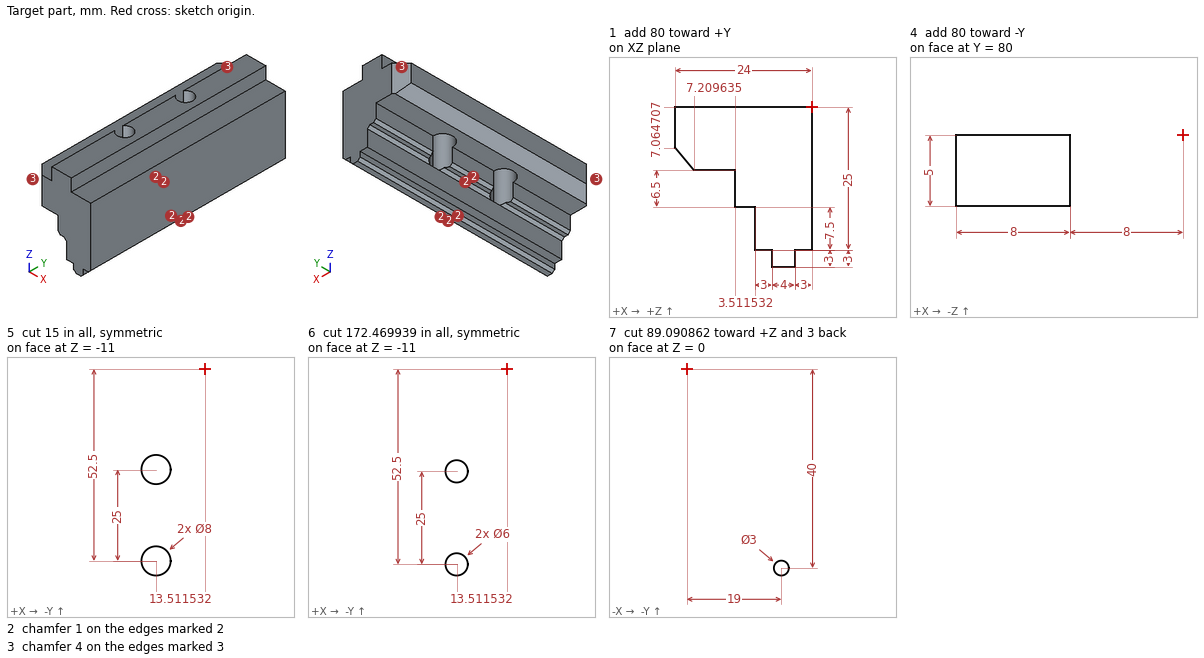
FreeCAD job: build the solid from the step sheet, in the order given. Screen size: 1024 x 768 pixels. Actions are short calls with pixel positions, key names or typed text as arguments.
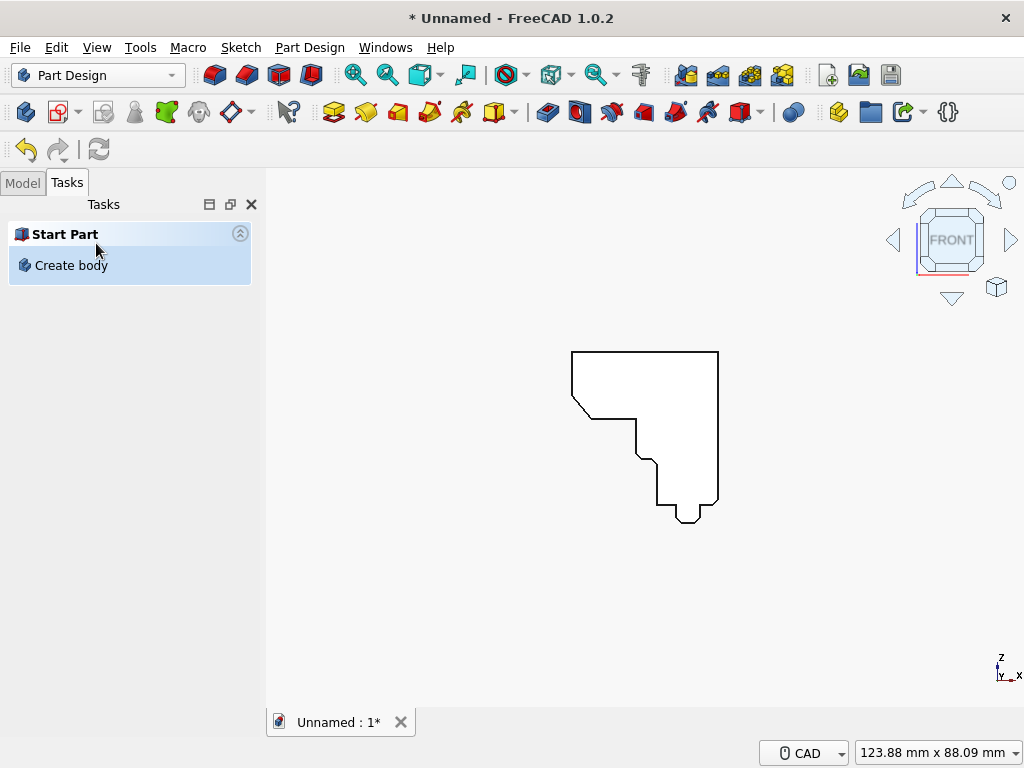
click(572, 372)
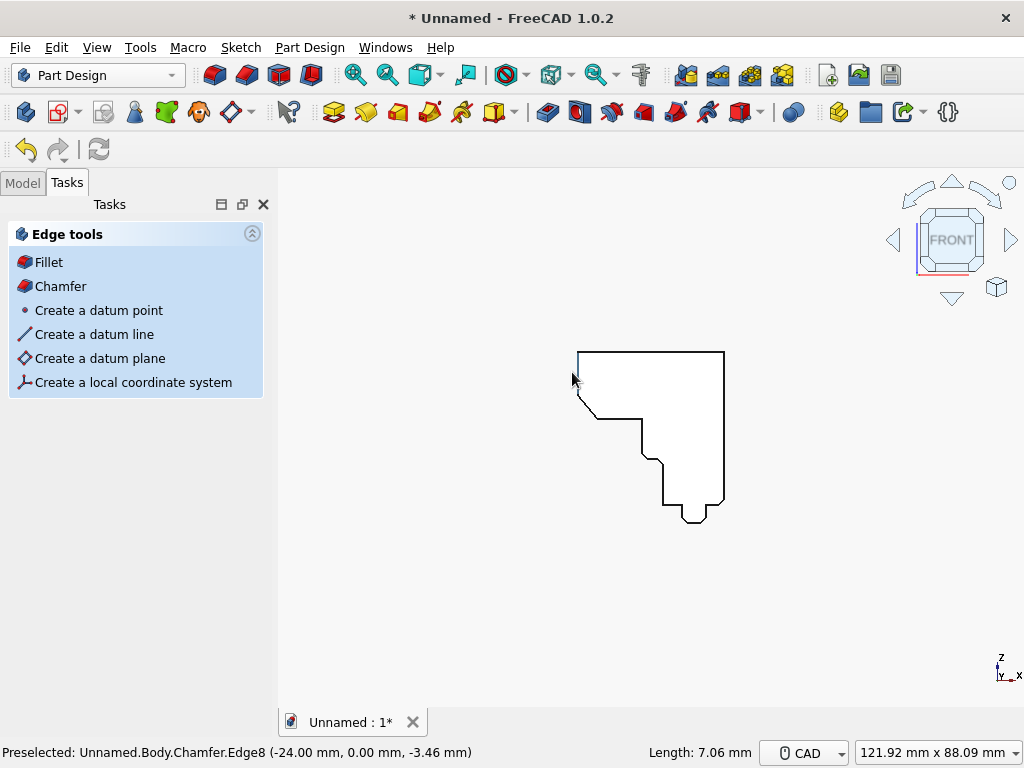
key(3)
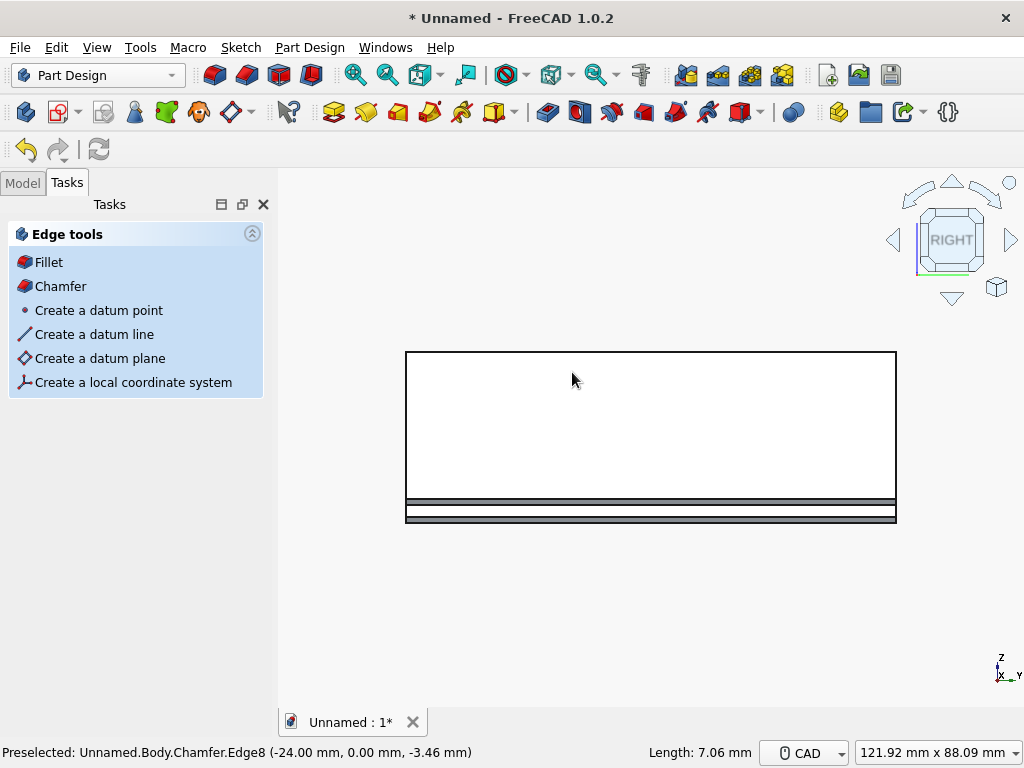
key(5)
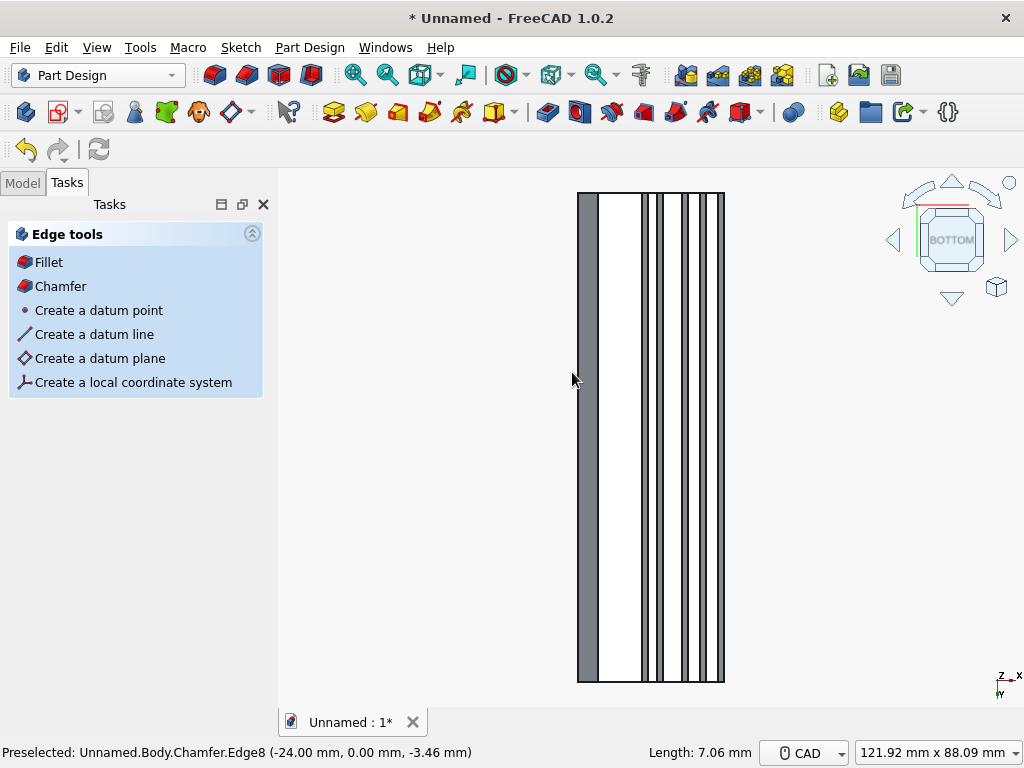
key(4)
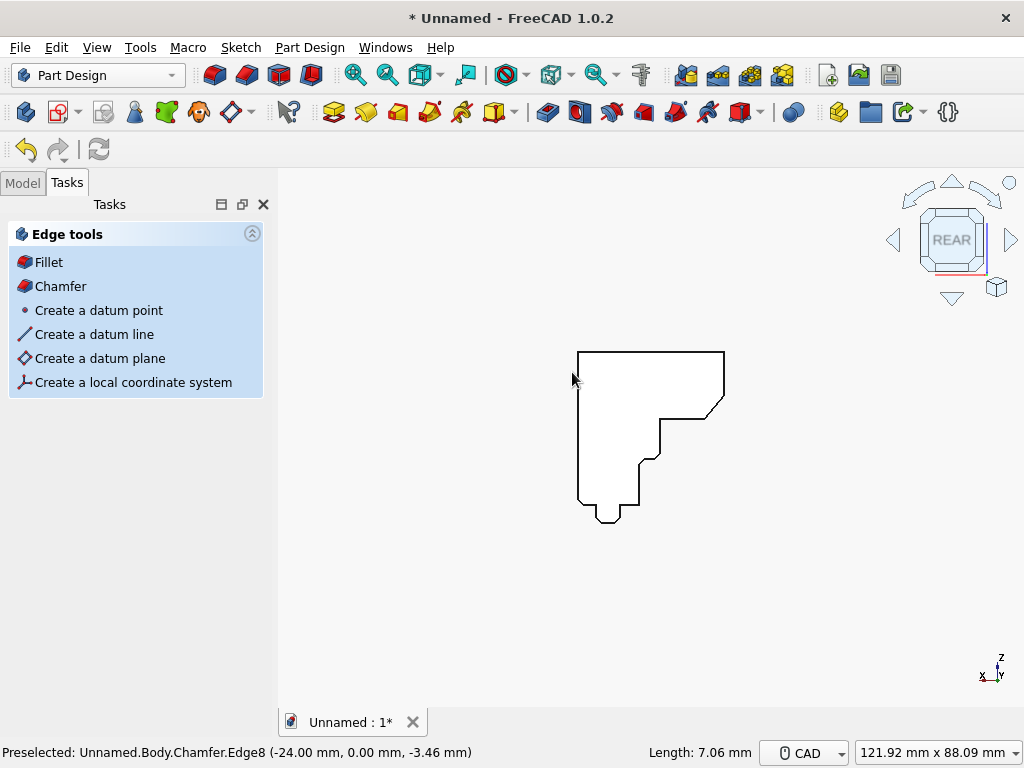
key(v)
key(f)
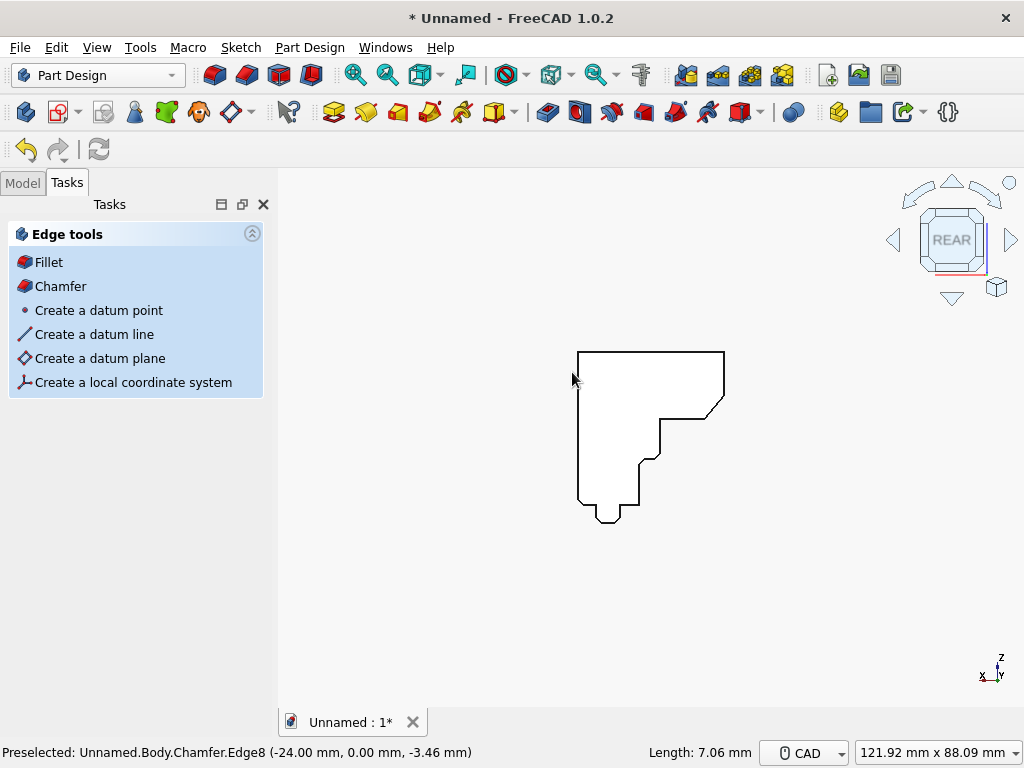
click(724, 372, ctrl)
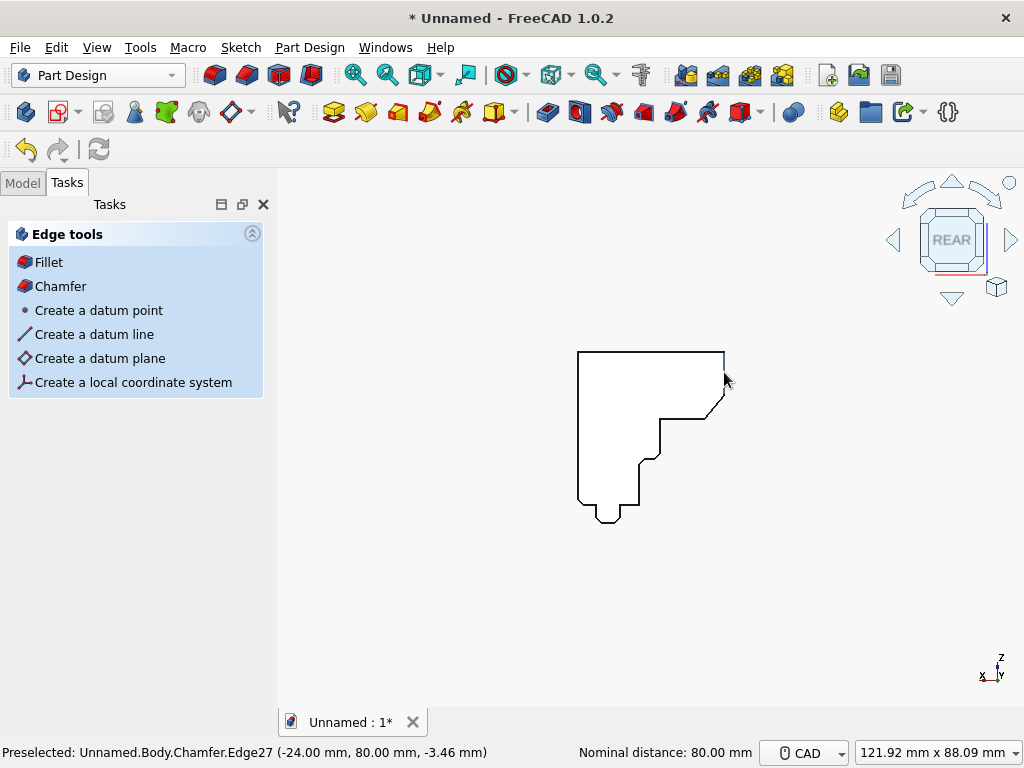
click(248, 76)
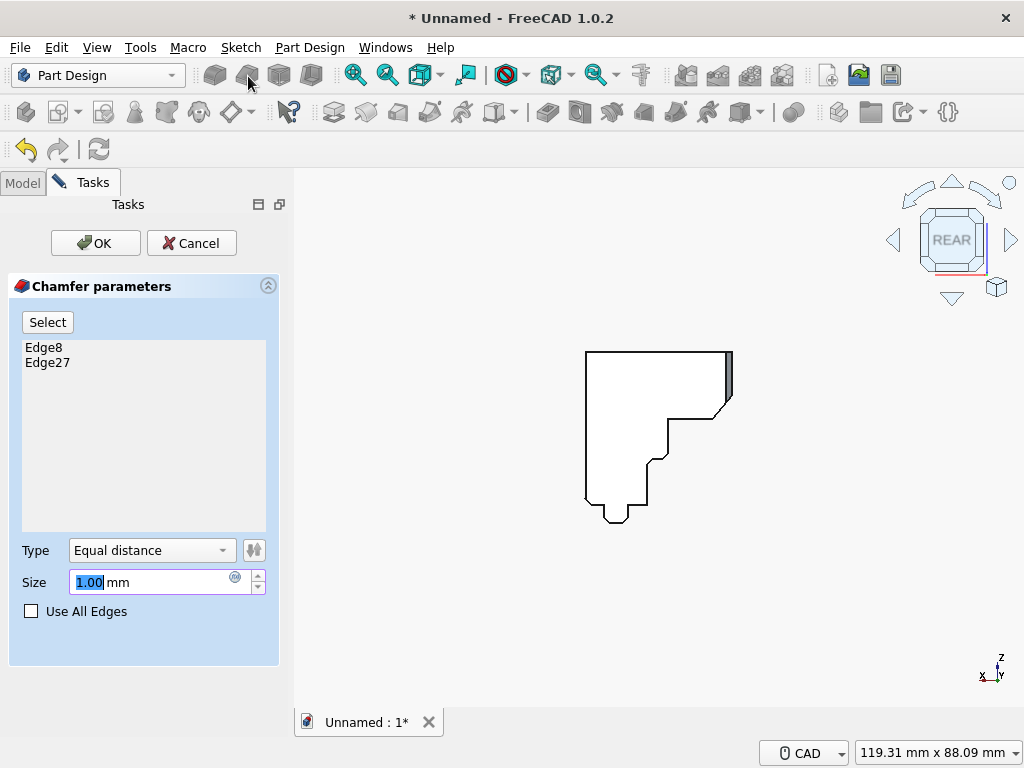
text(4)
key(Tab)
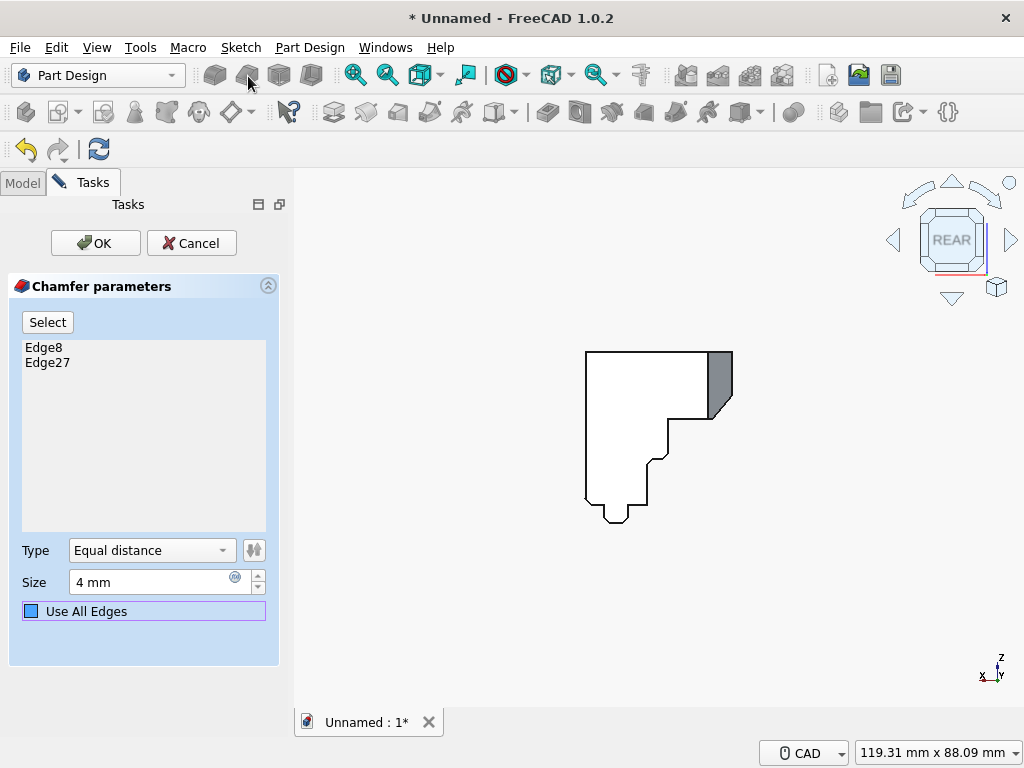
click(96, 243)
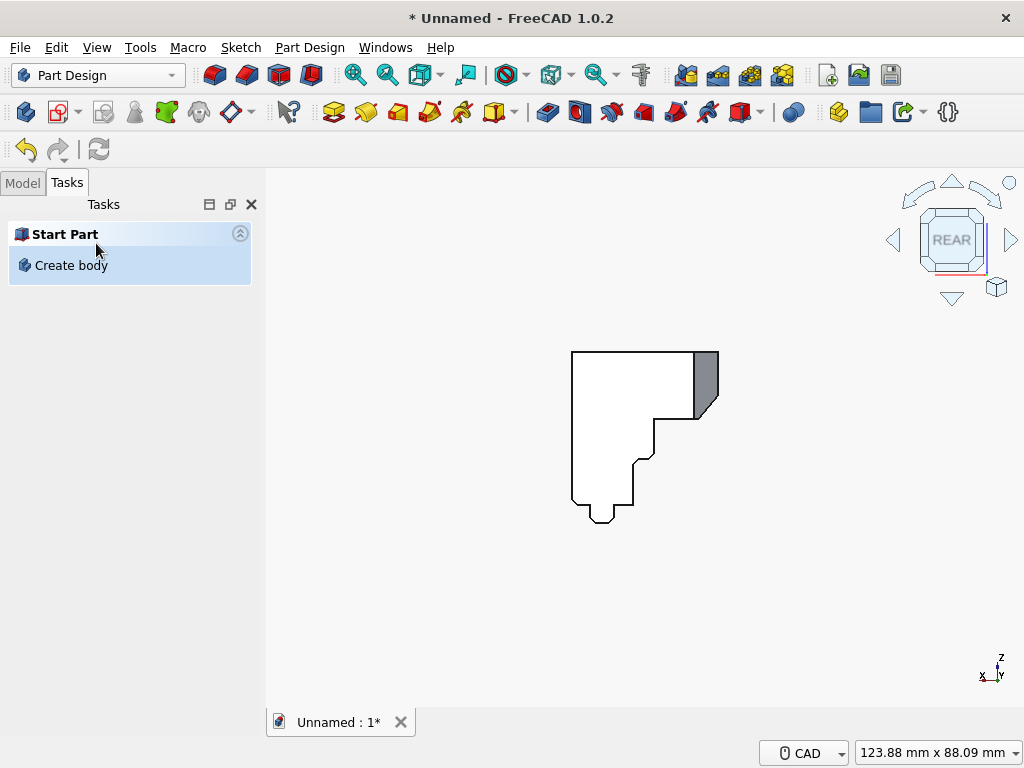
key(v)
key(f)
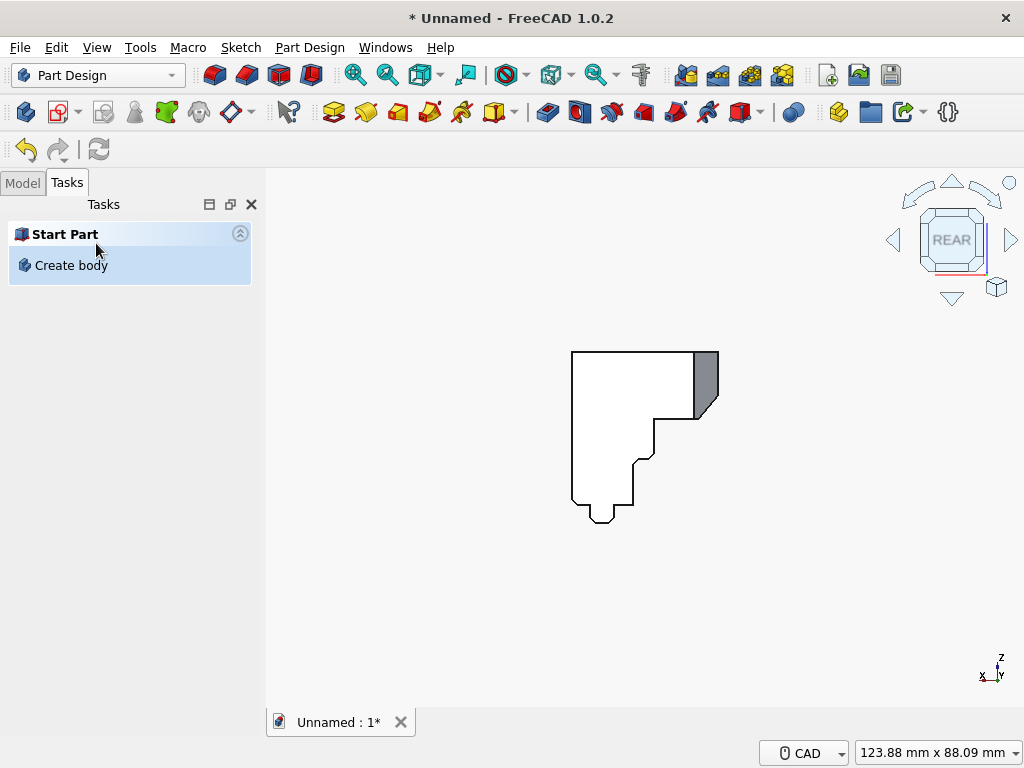
click(615, 412)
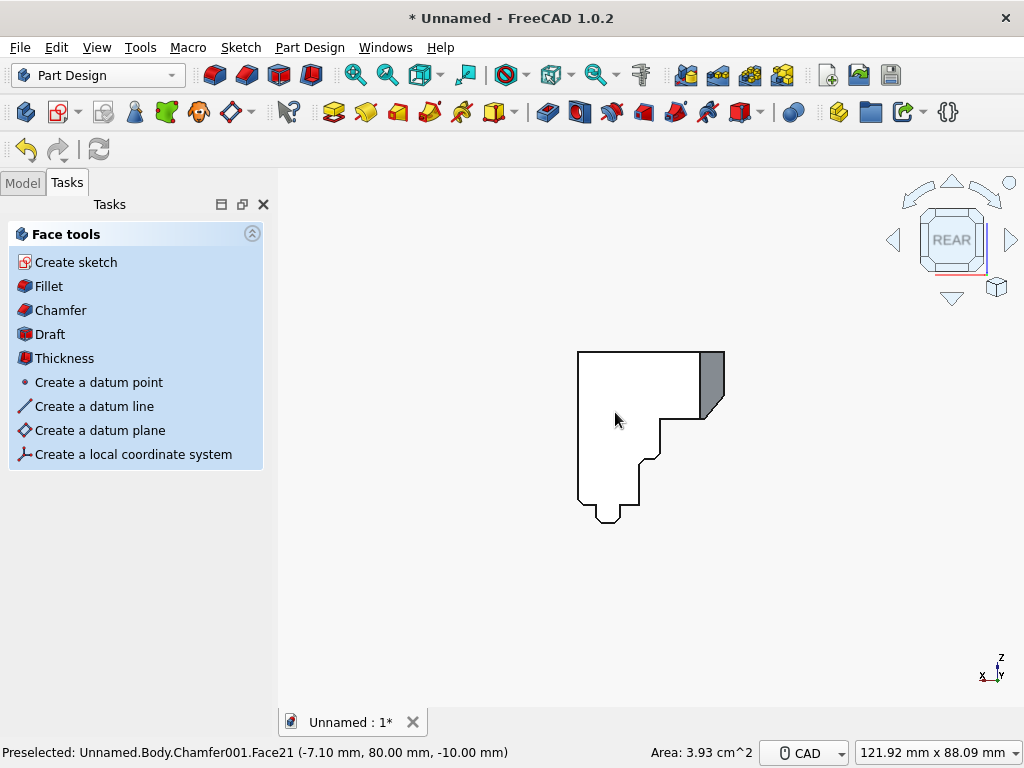
click(58, 112)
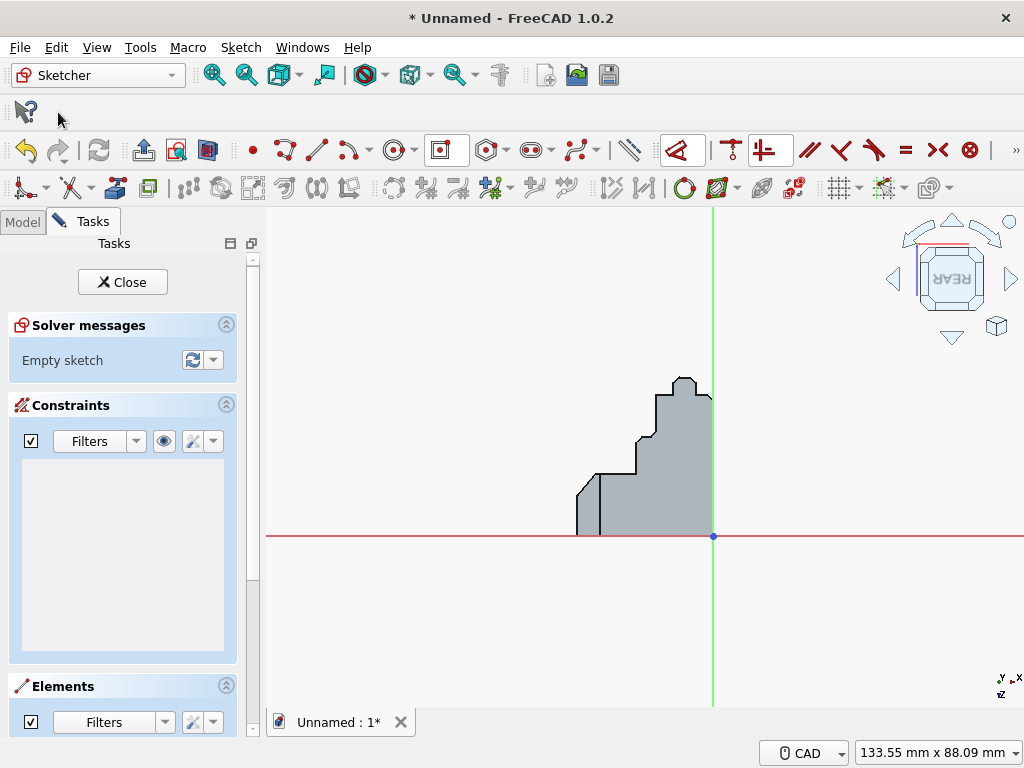
scroll(698, 581, up, 7)